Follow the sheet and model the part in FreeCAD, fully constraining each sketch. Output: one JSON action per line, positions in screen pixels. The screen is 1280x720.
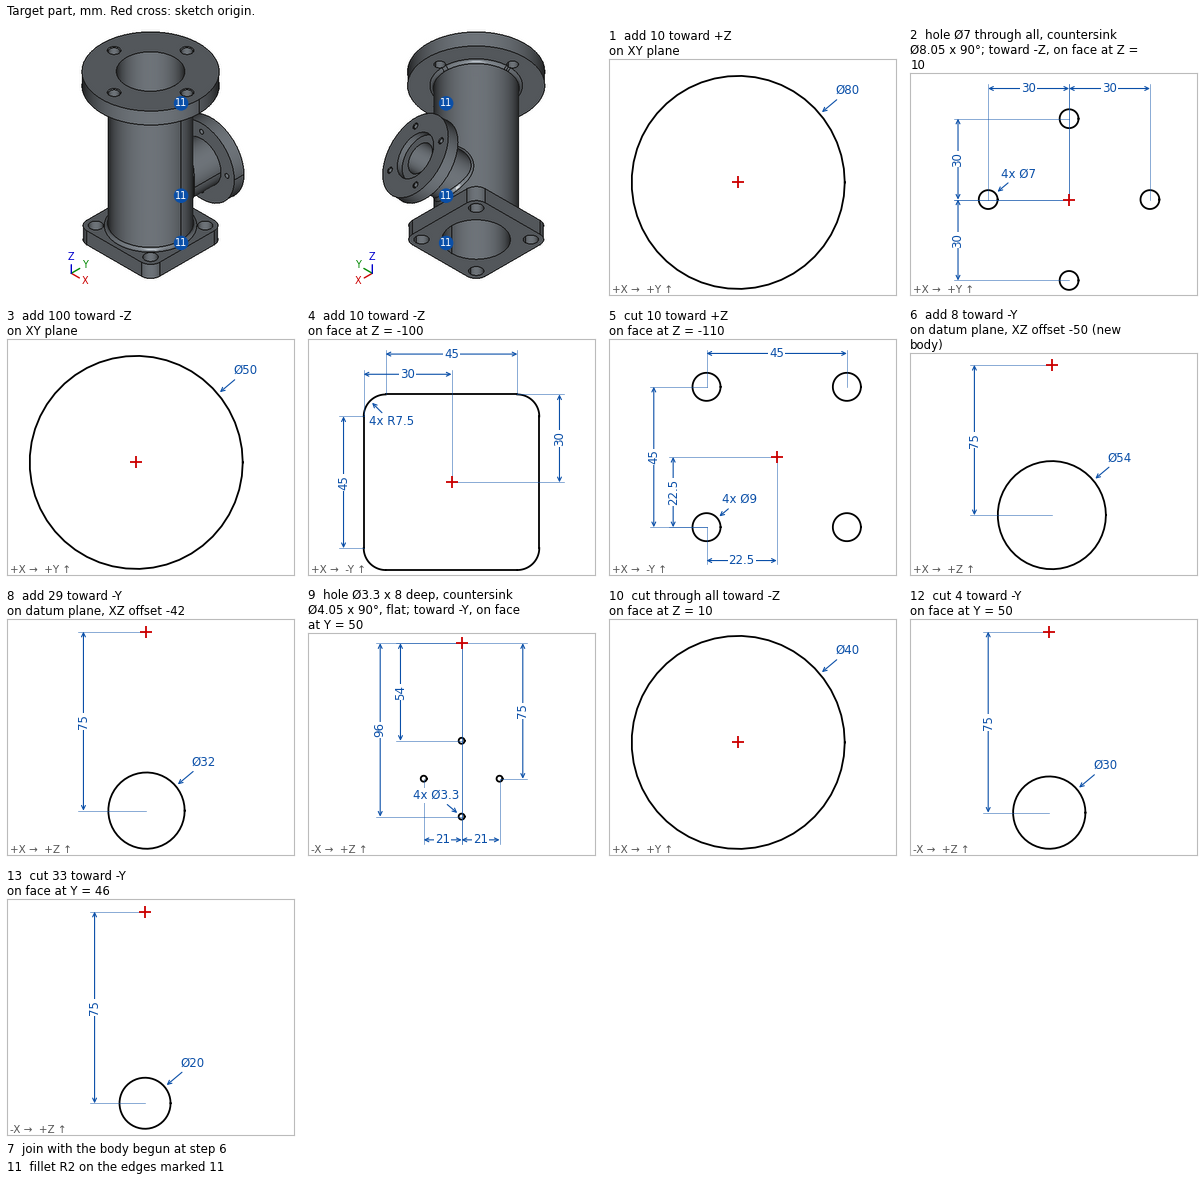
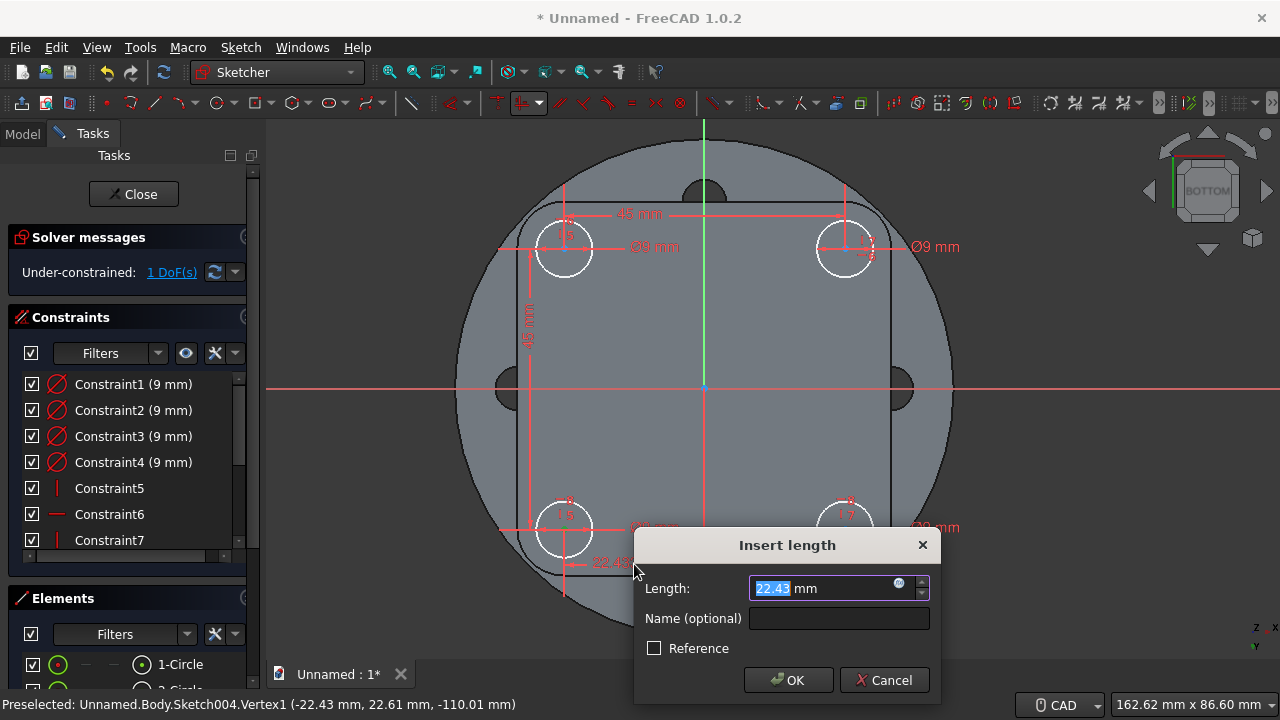
{"action": "type", "text": "22.5"}
{"action": "key", "text": "Return"}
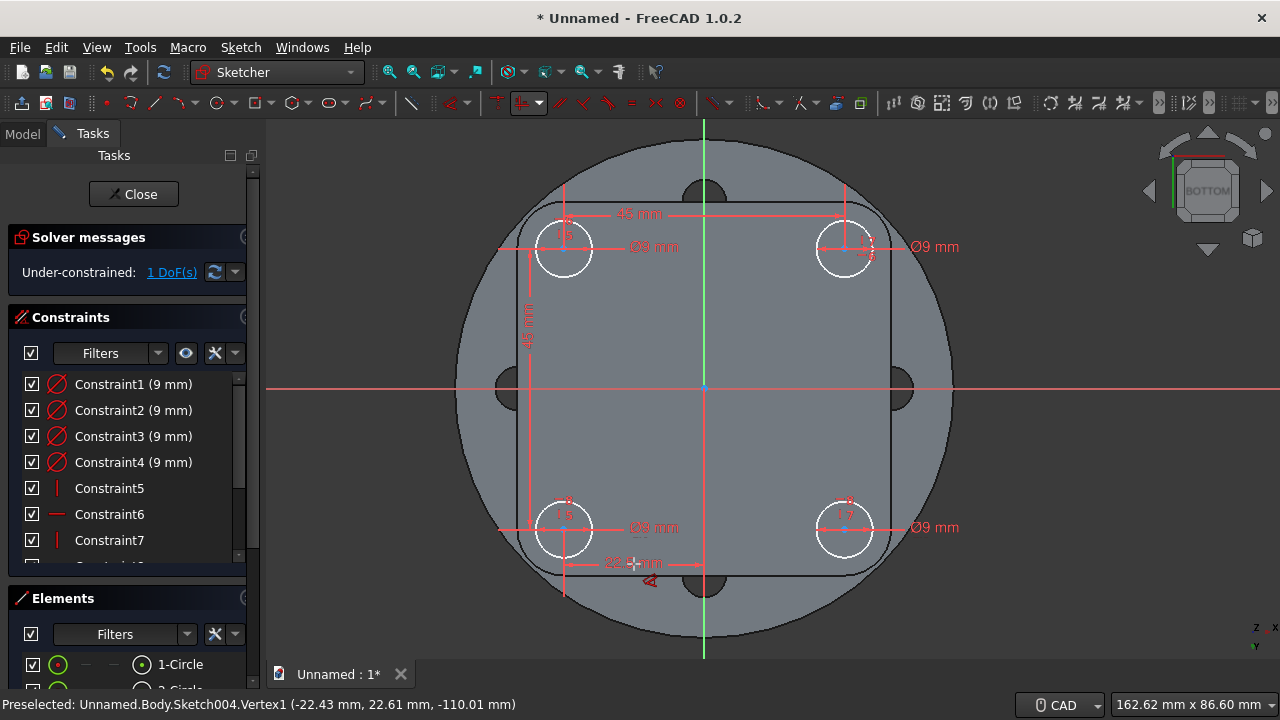
{"action": "left_click", "coordinate": [564, 530]}
{"action": "left_click", "coordinate": [530, 459]}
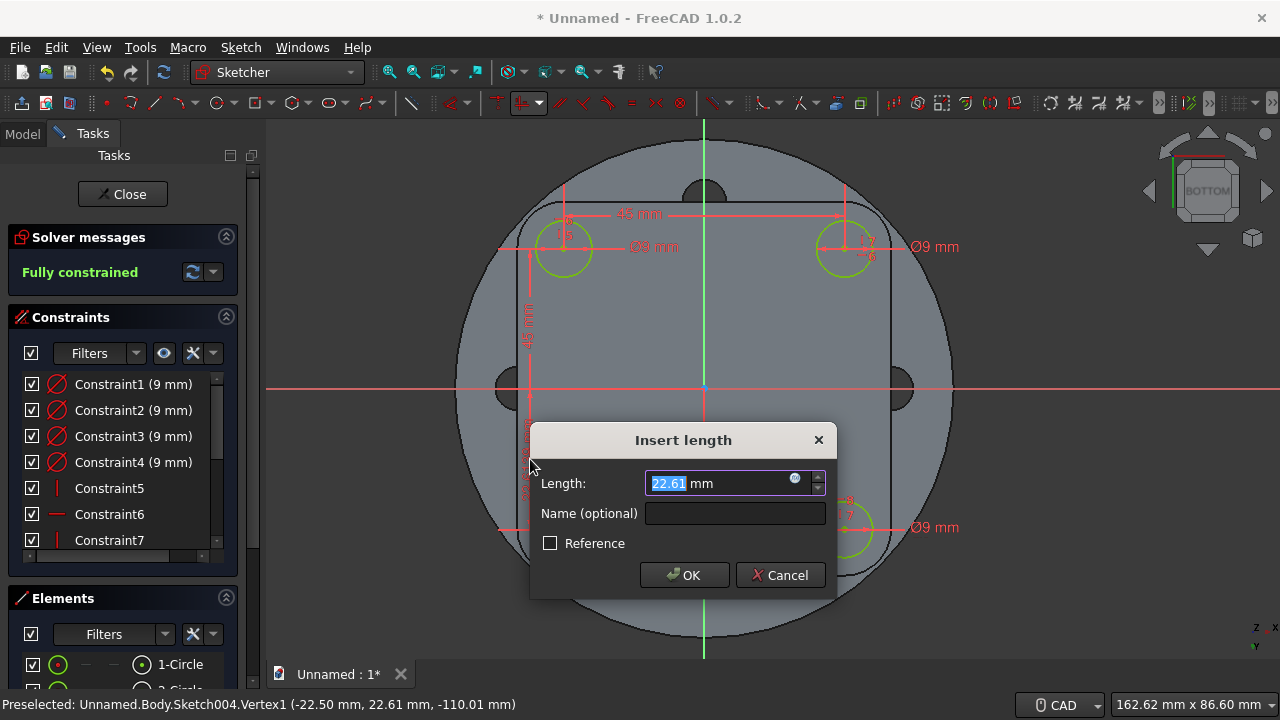
{"action": "type", "text": "22.5"}
{"action": "key", "text": "Return"}
{"action": "key", "text": "Escape"}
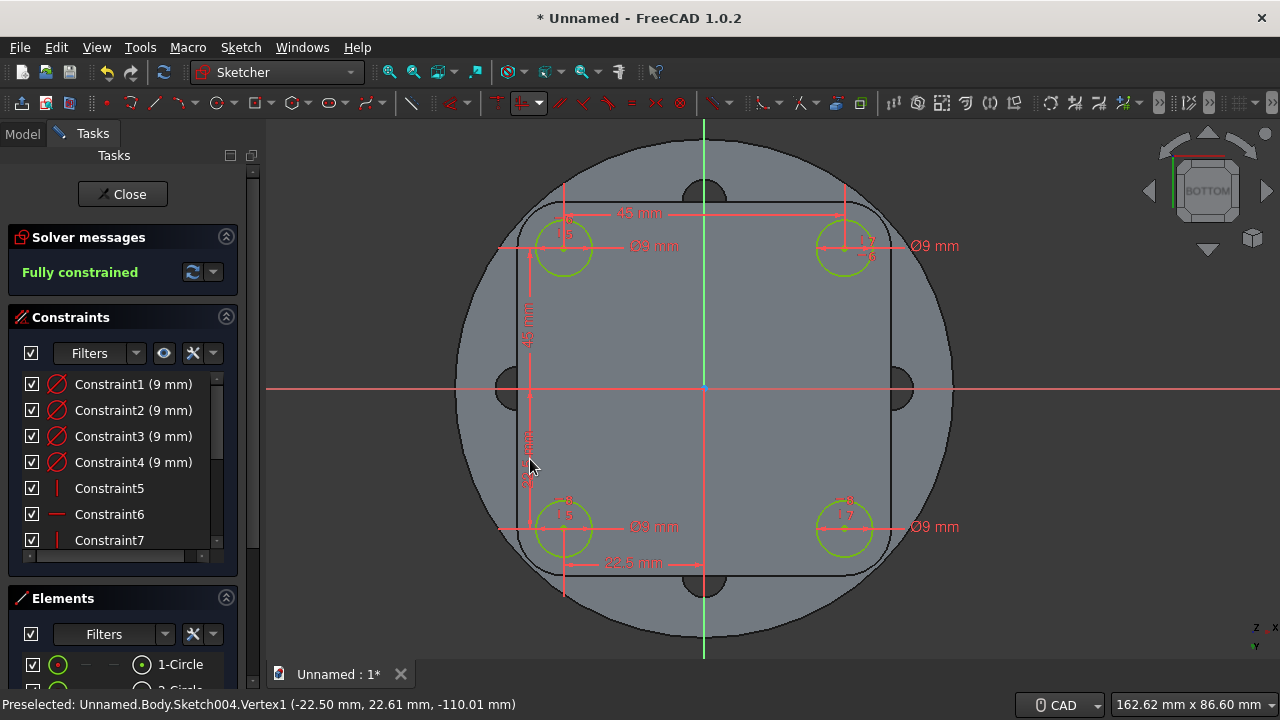
{"action": "left_click", "coordinate": [123, 194]}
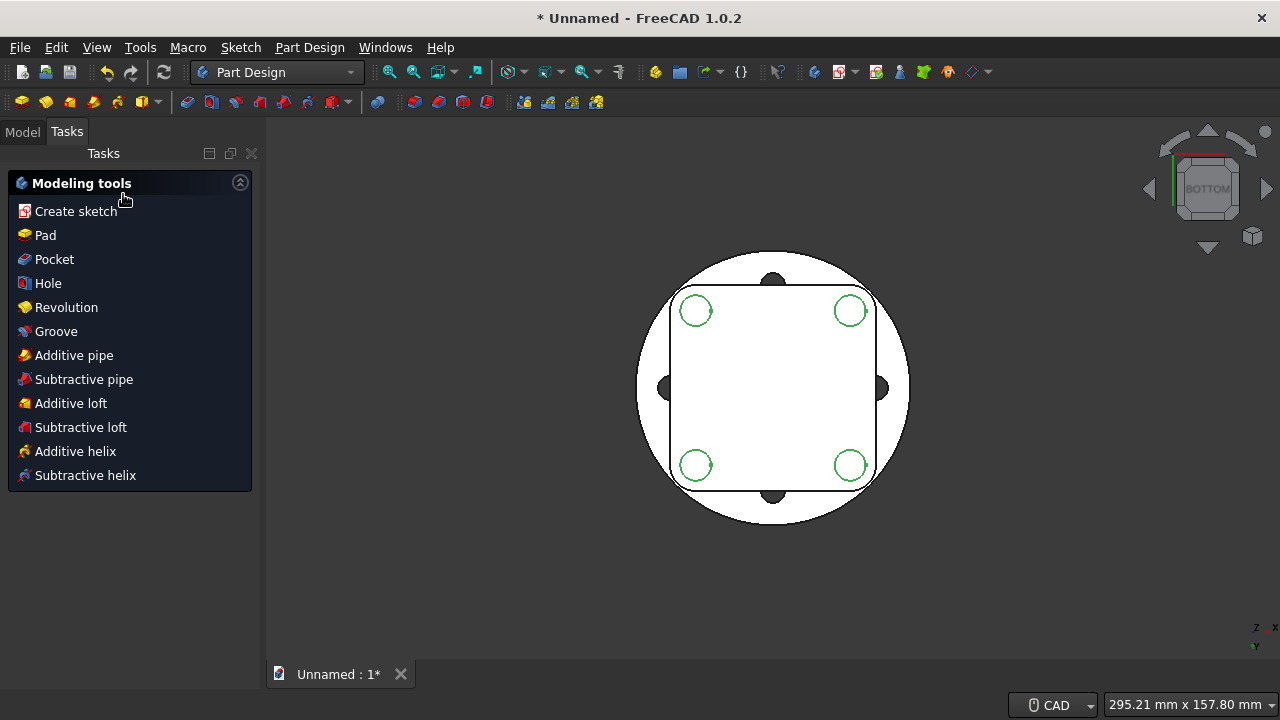
{"action": "left_click", "coordinate": [188, 102]}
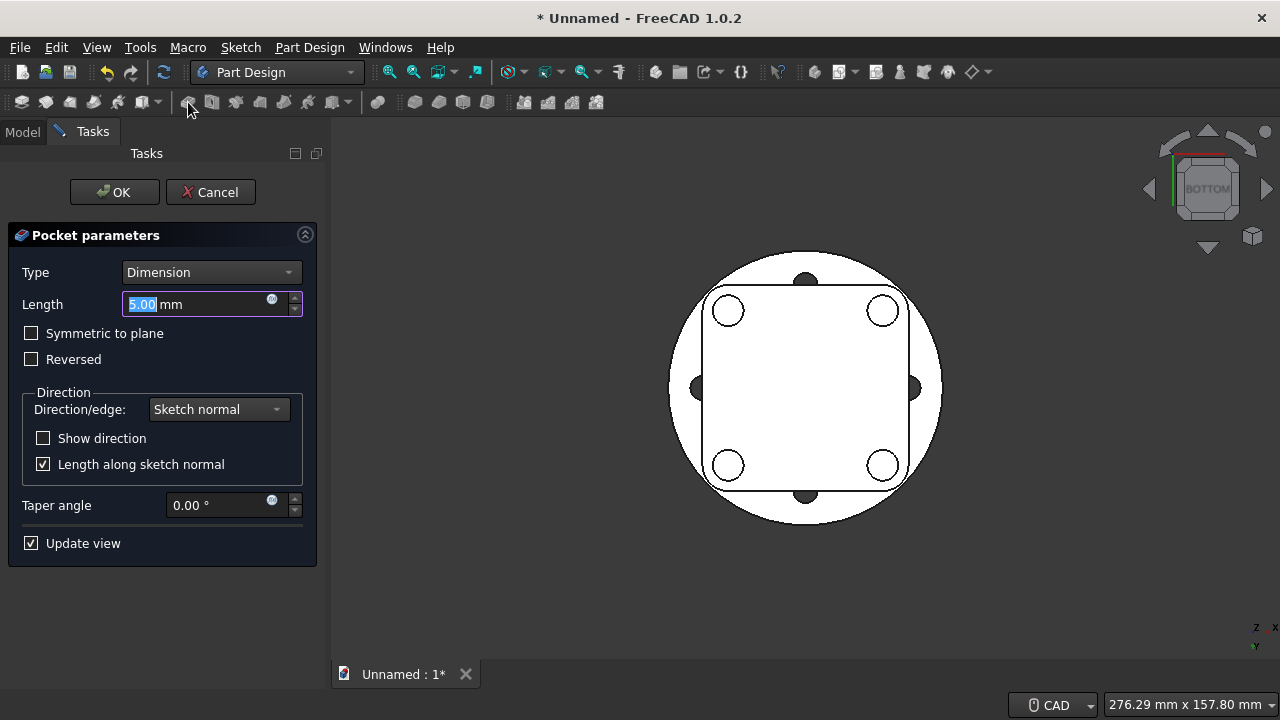
{"action": "type", "text": "10"}
{"action": "key", "text": "Tab"}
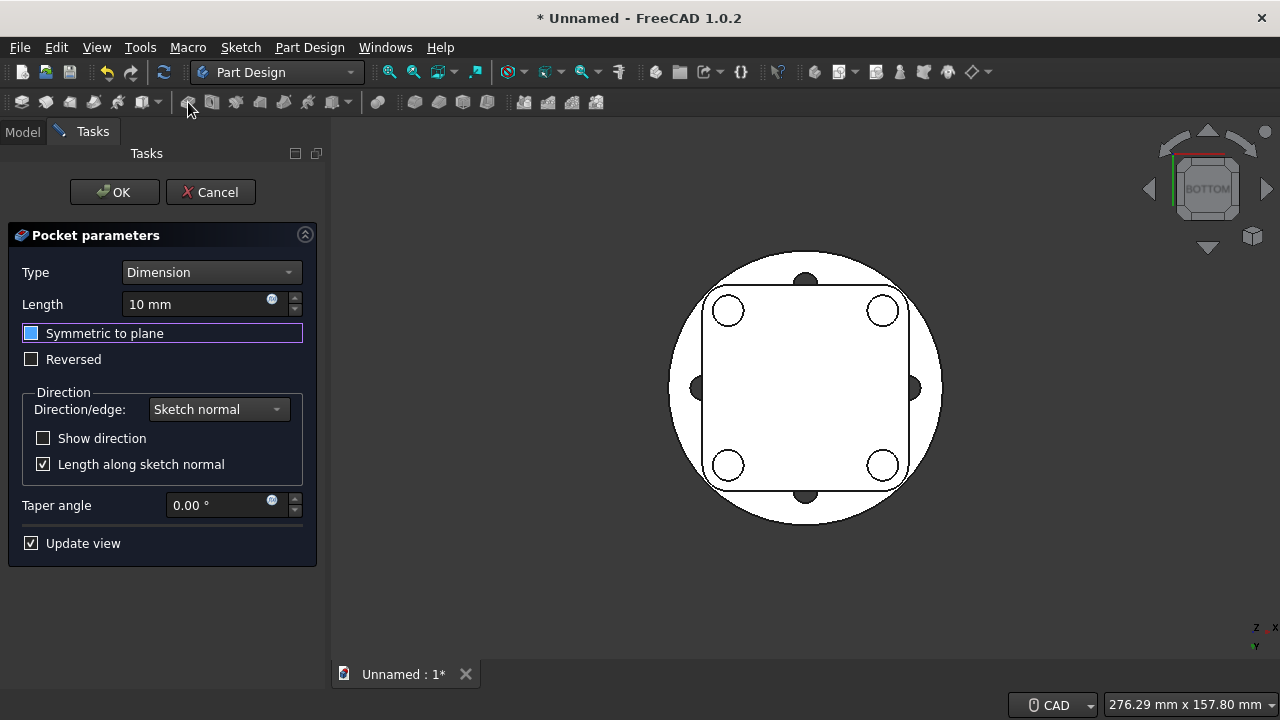
{"action": "left_click", "coordinate": [115, 192]}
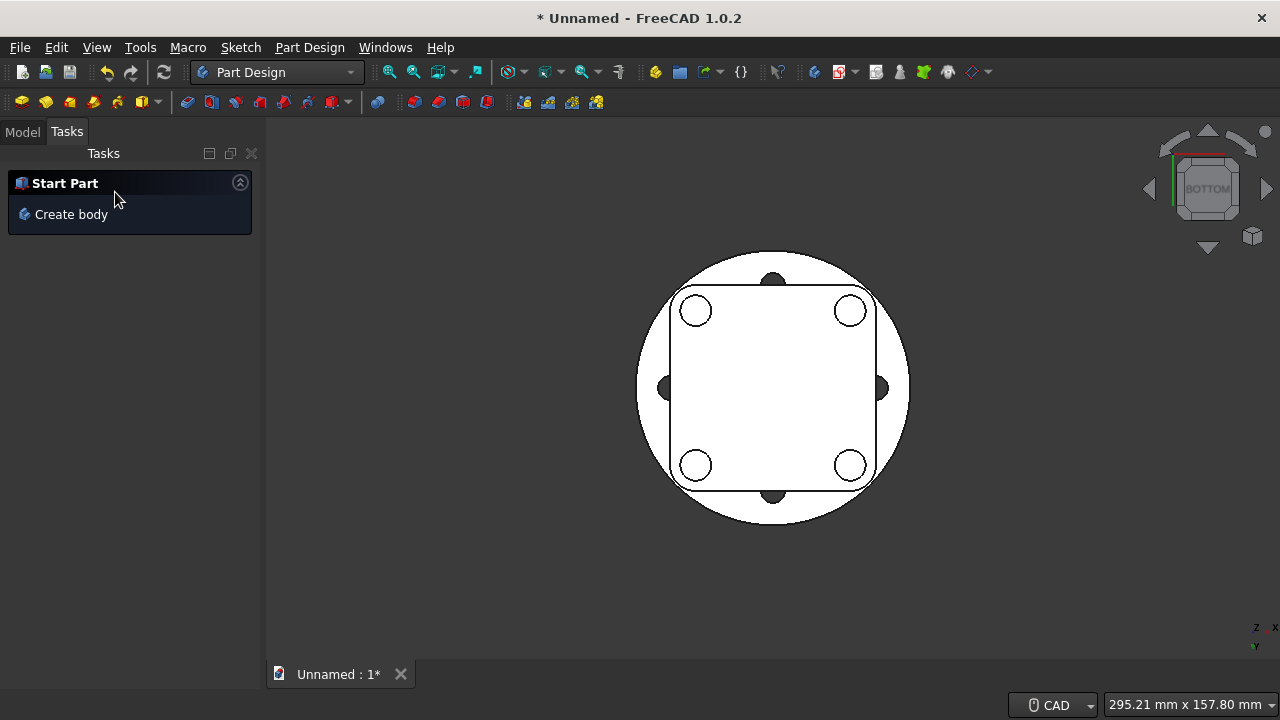
{"action": "left_click", "coordinate": [816, 72]}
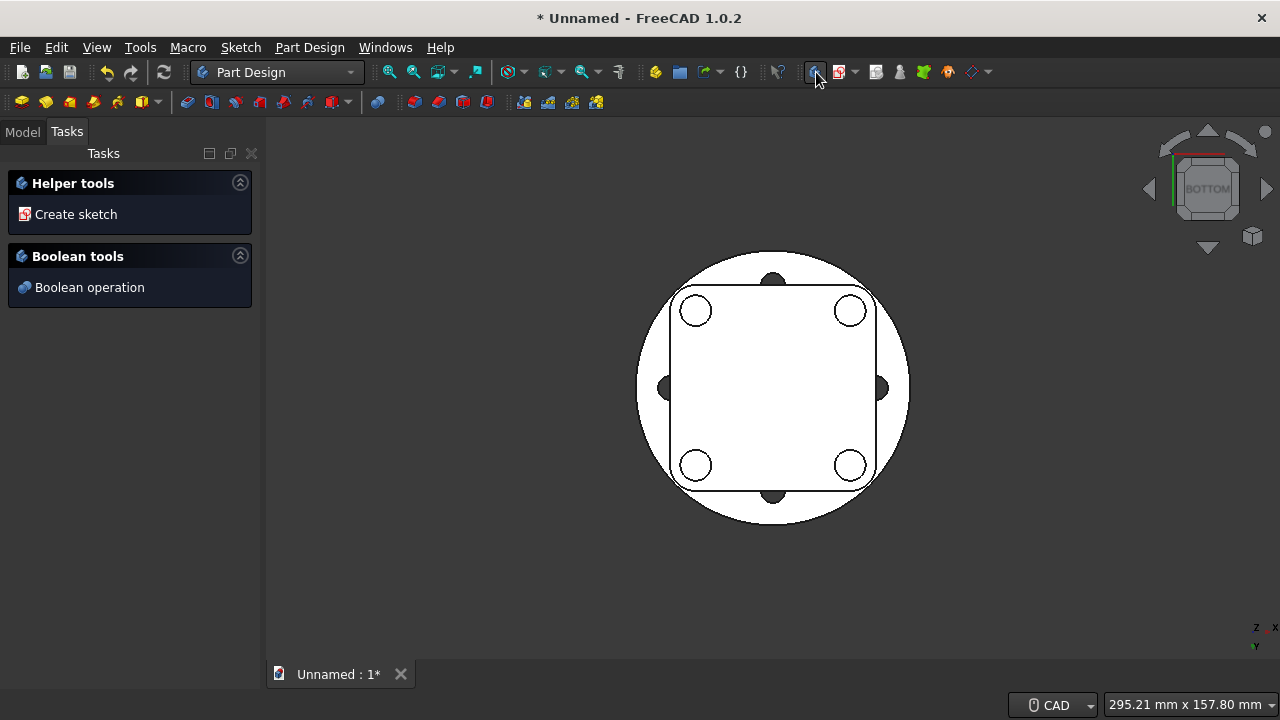
{"action": "left_click", "coordinate": [23, 131]}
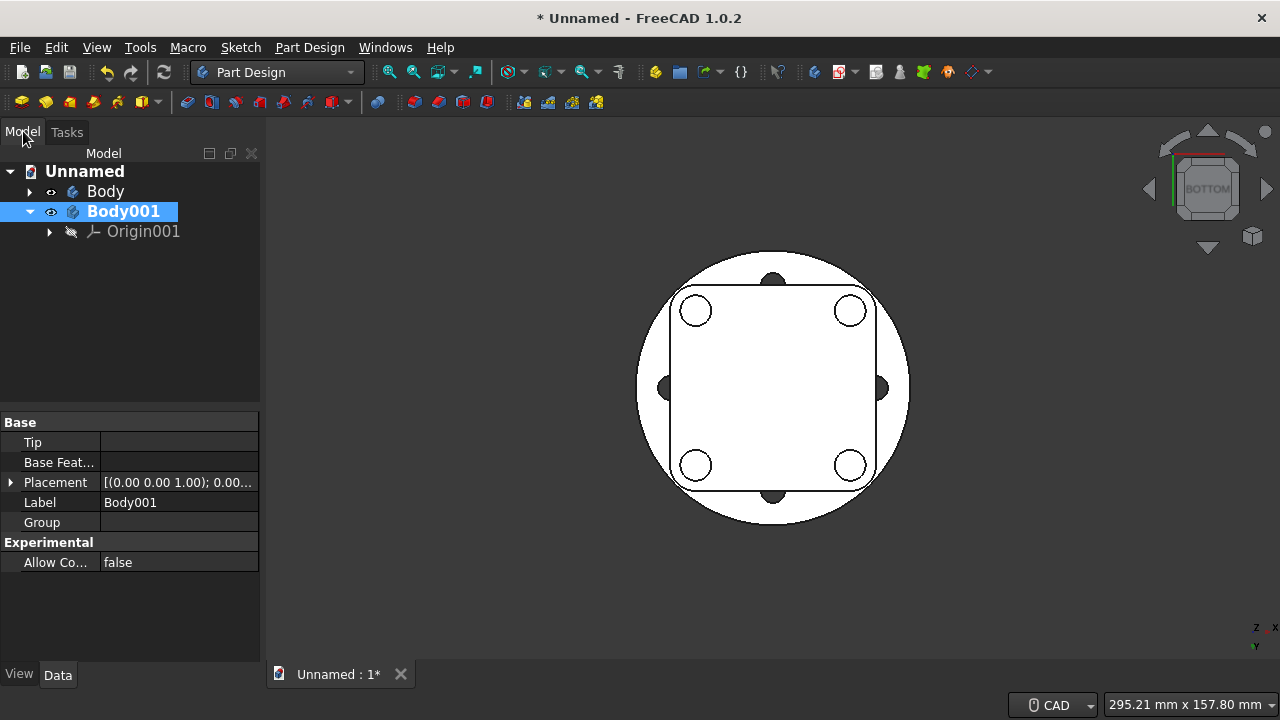
{"action": "left_click", "coordinate": [50, 232]}